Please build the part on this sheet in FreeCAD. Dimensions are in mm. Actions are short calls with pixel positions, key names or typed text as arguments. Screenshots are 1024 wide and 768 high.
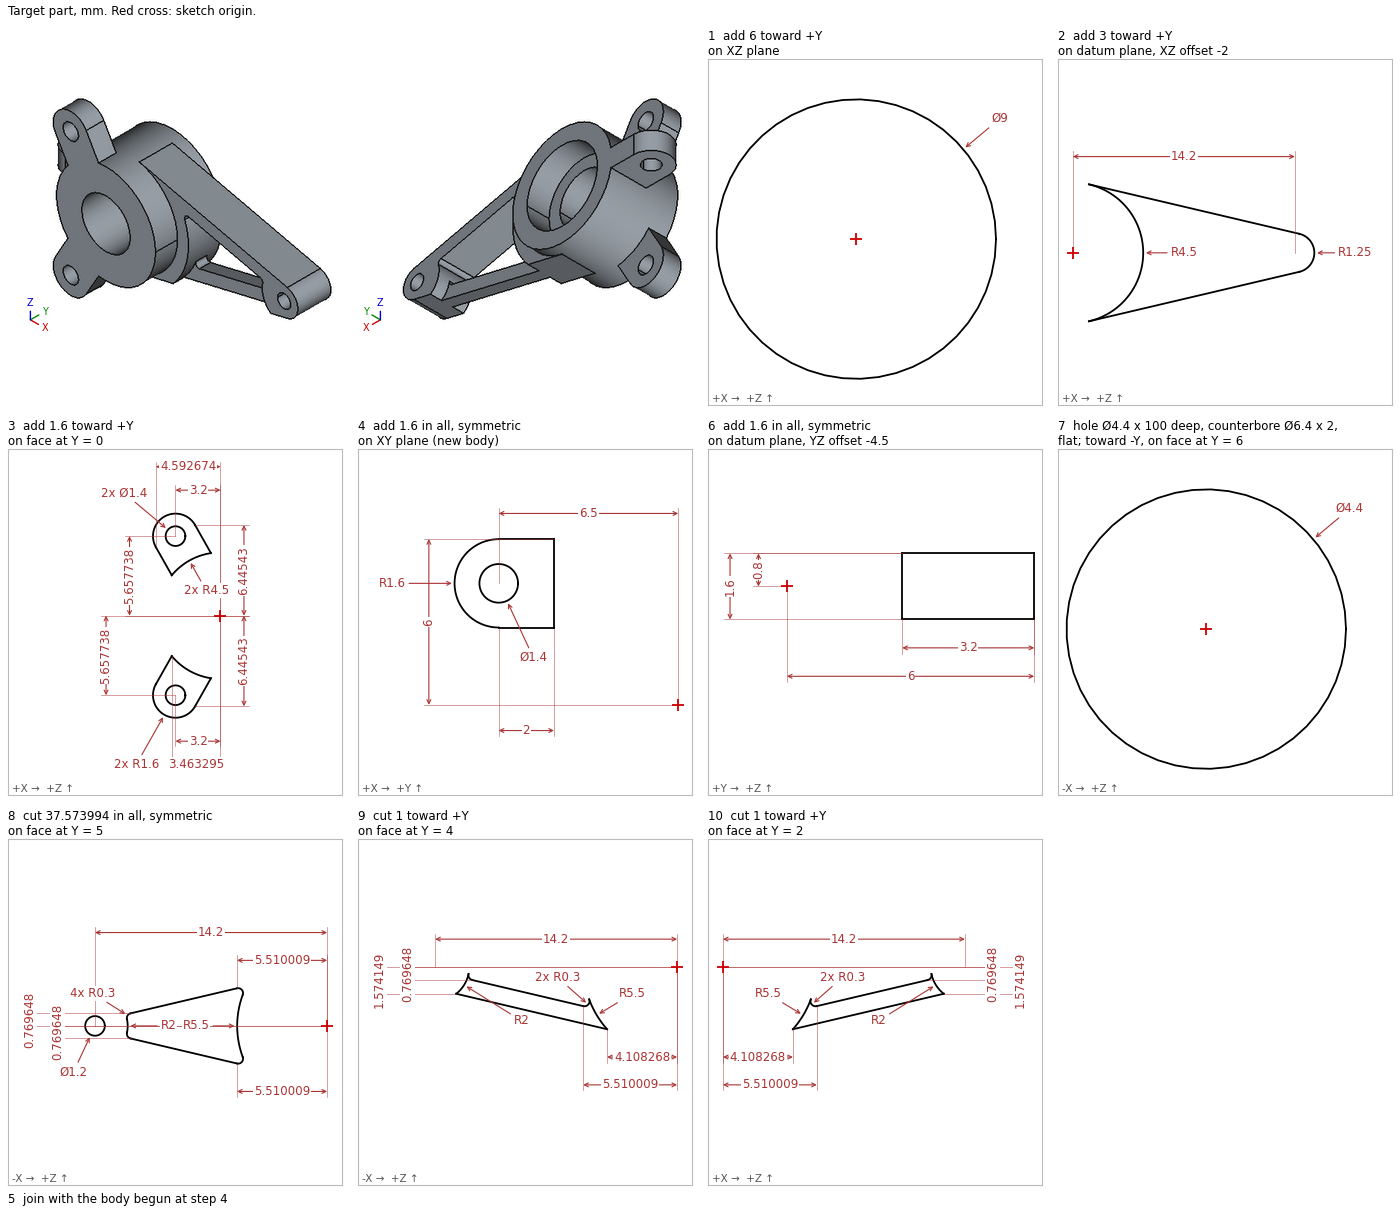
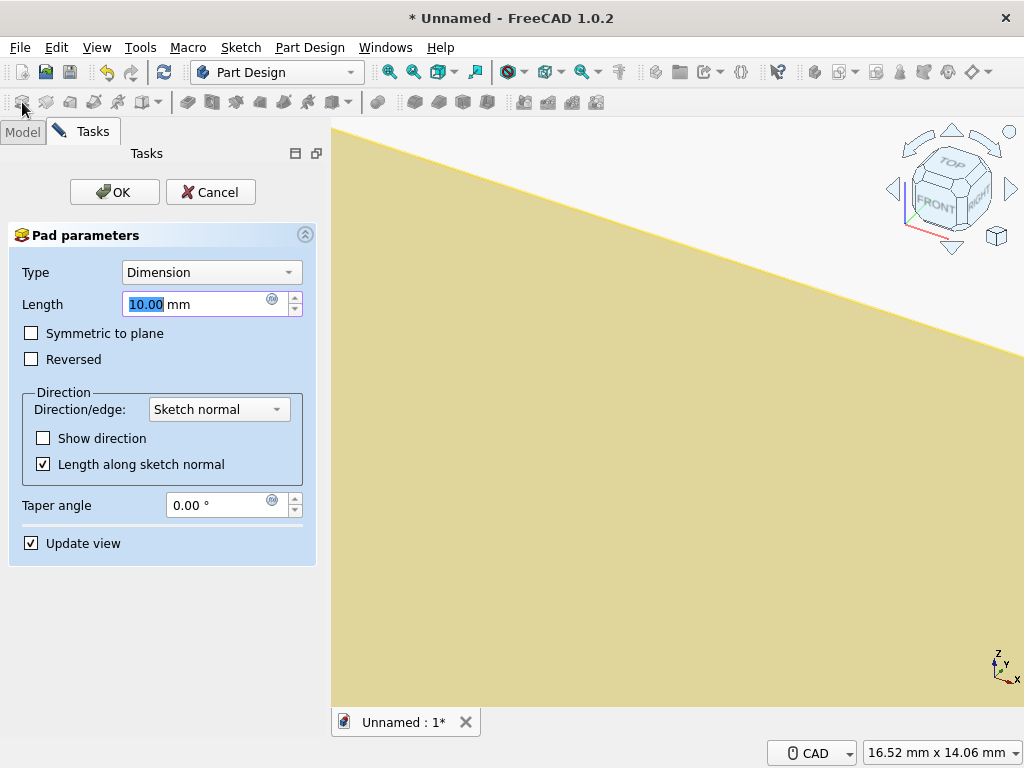
text(3)
key(Tab)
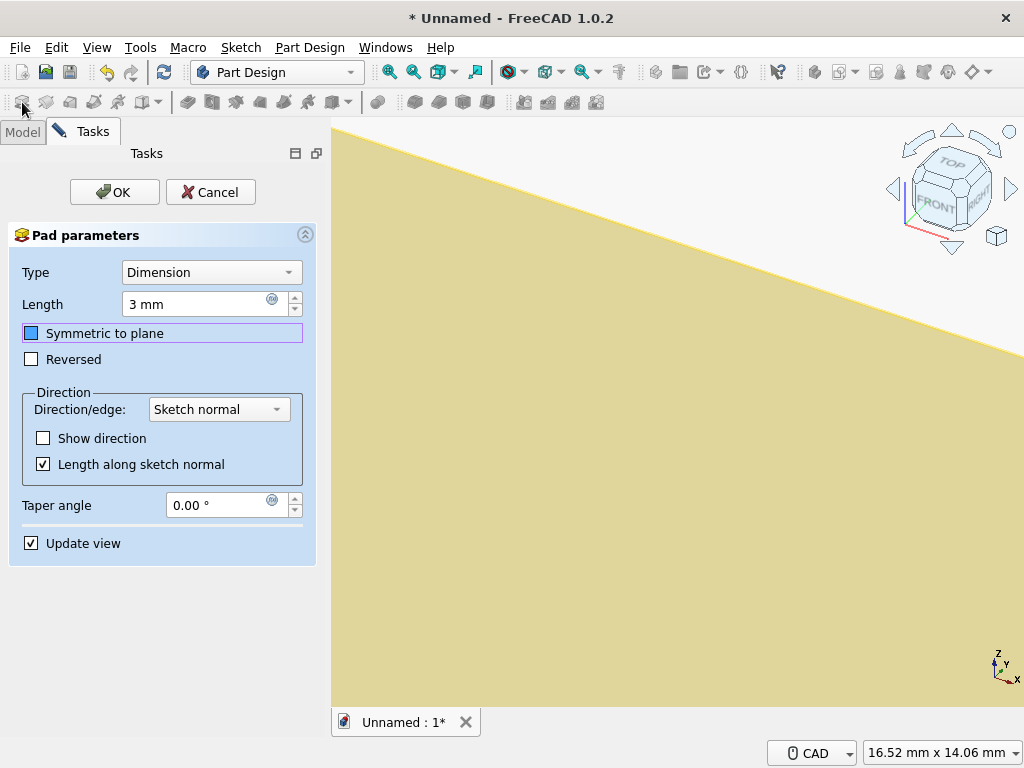
click(30, 359)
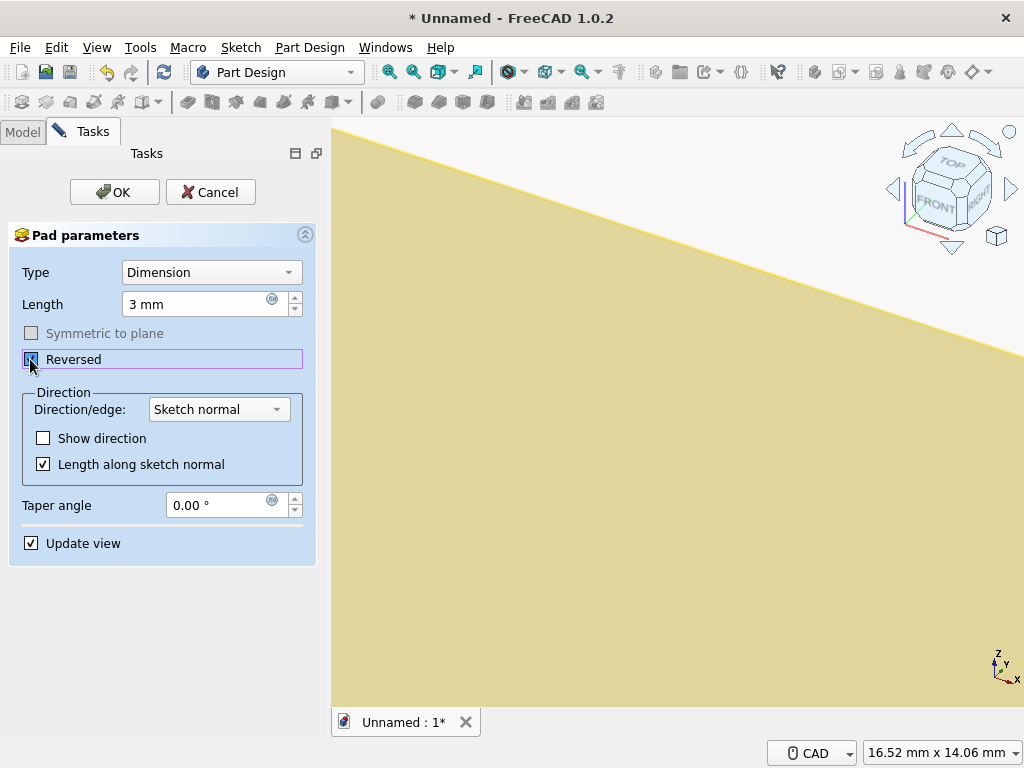
click(115, 192)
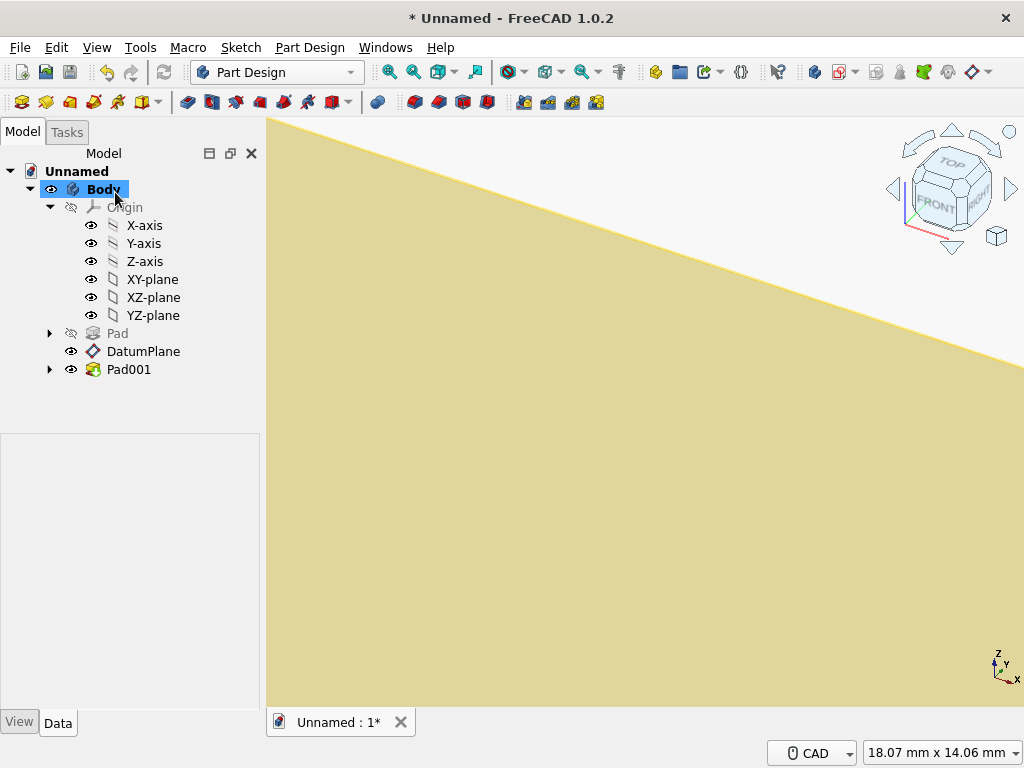
click(116, 351)
key(space)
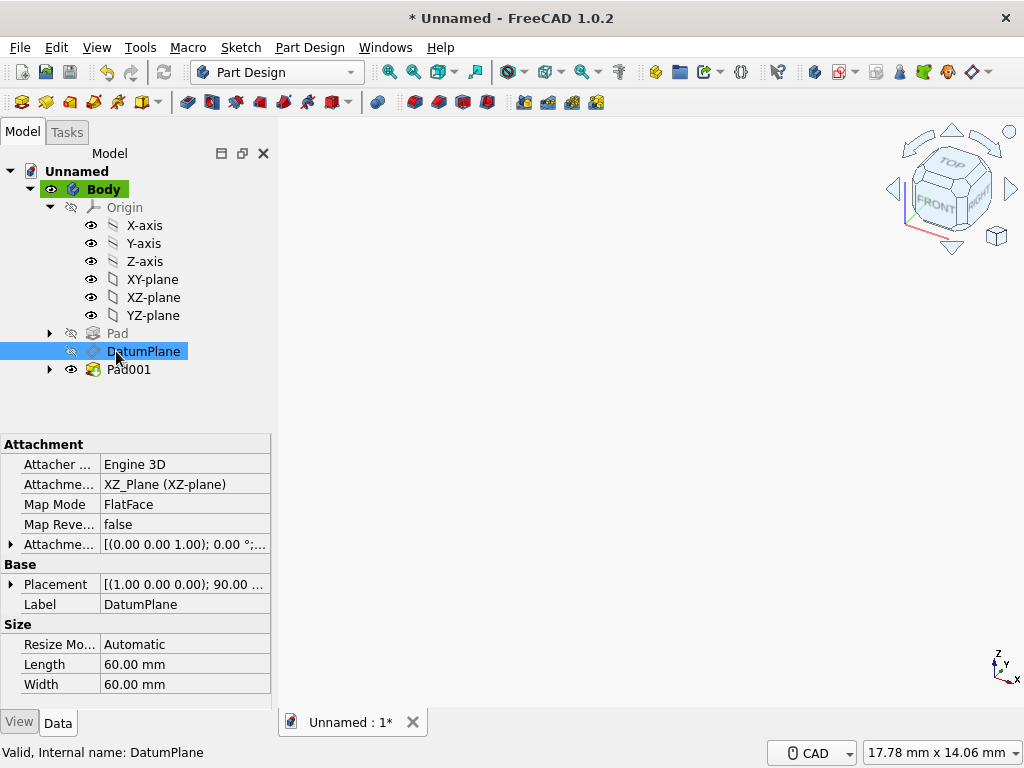
key(v)
key(f)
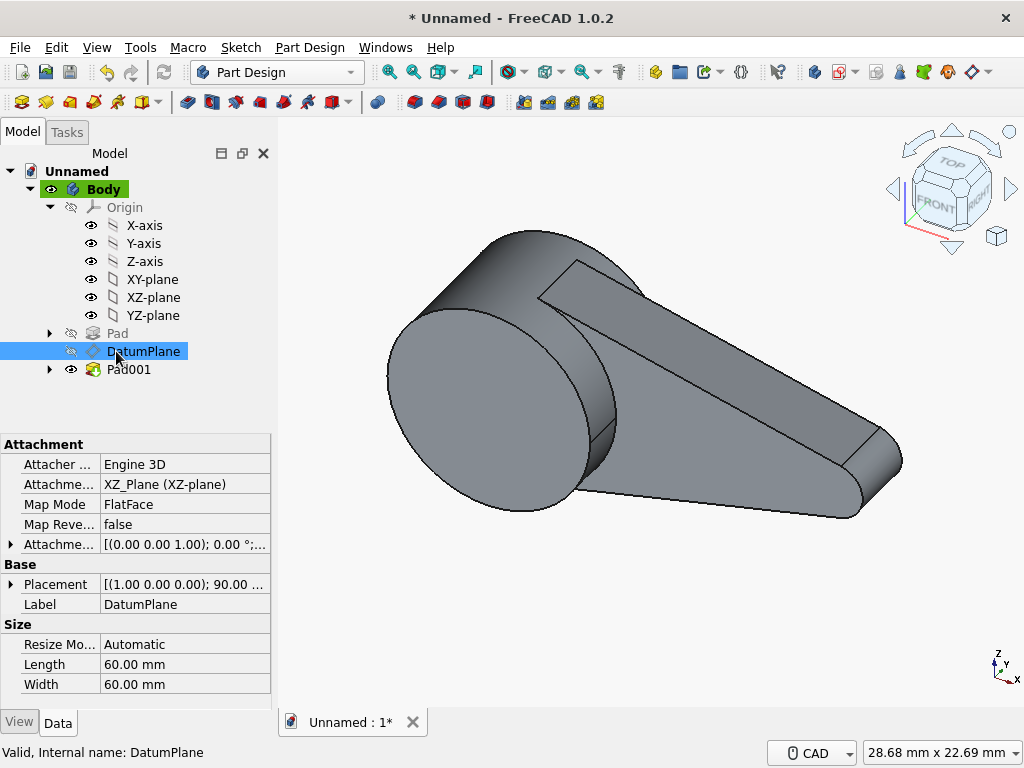
click(489, 409)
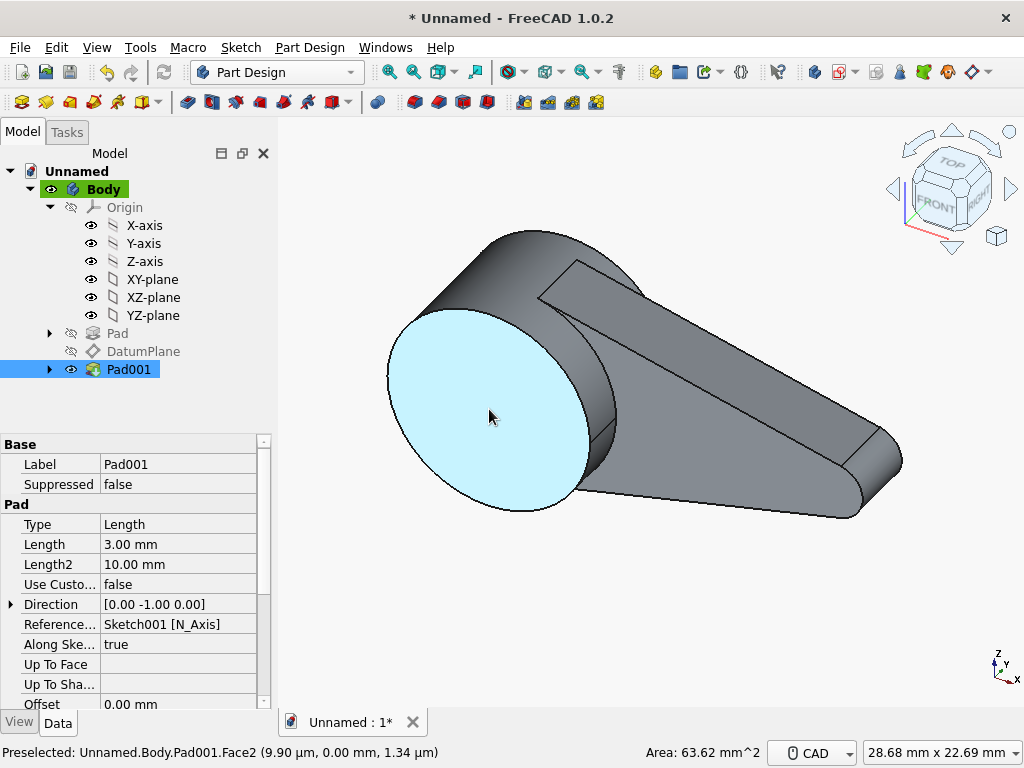
click(840, 72)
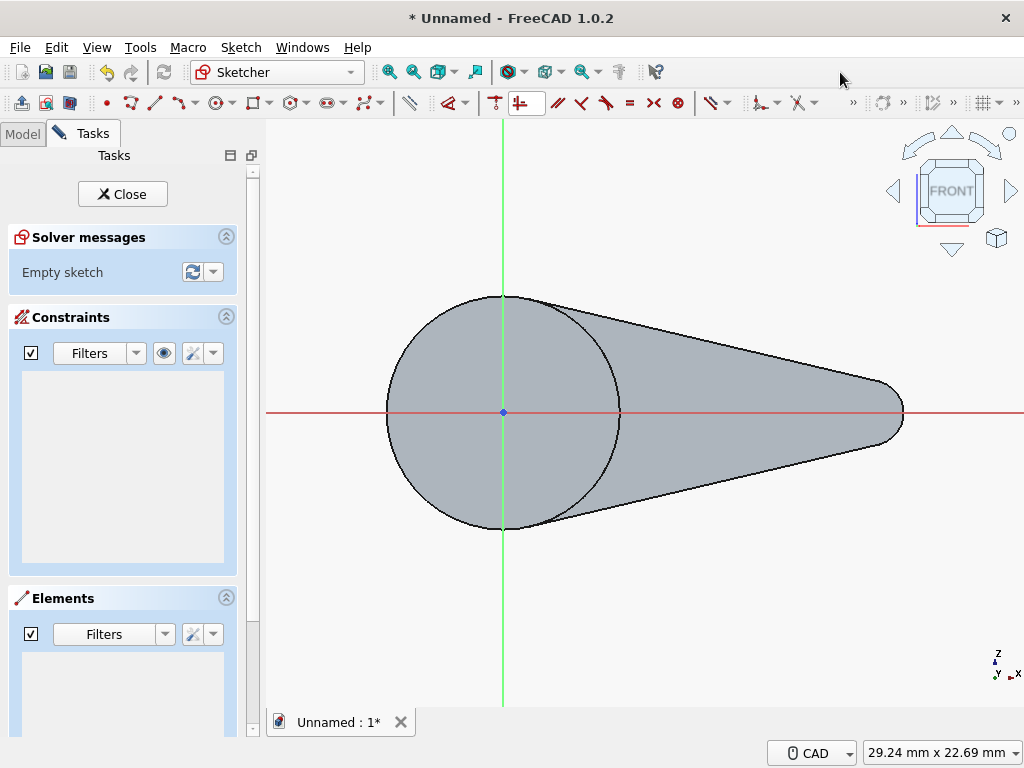
key(g)
key(l)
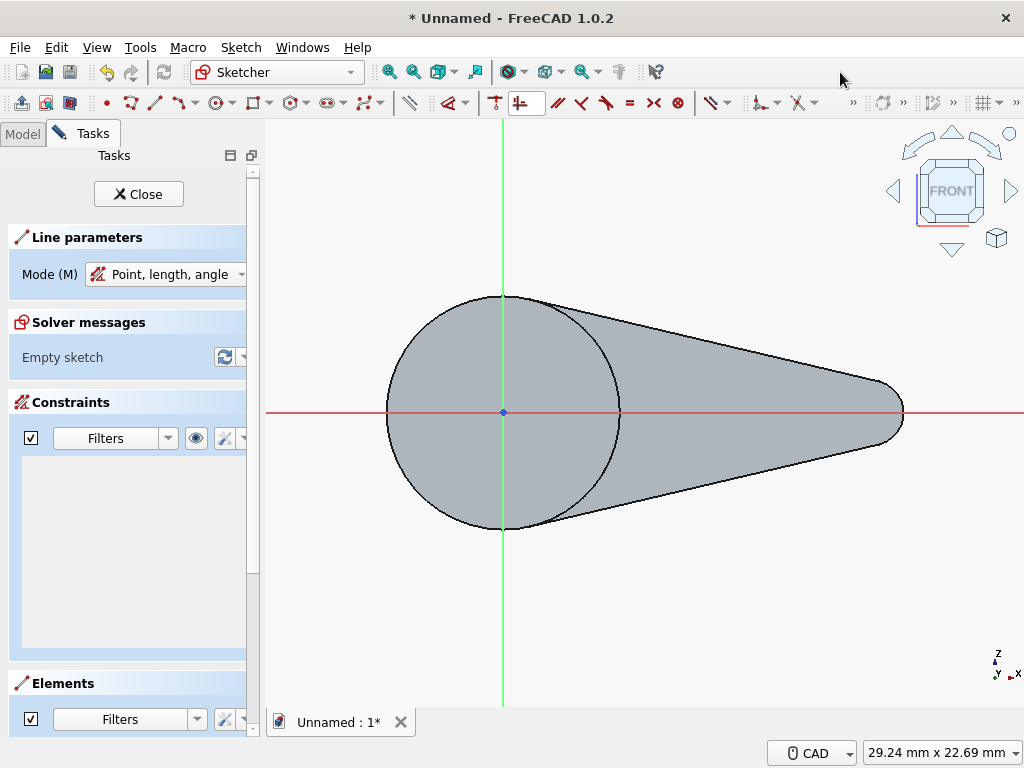
click(486, 298)
click(456, 246)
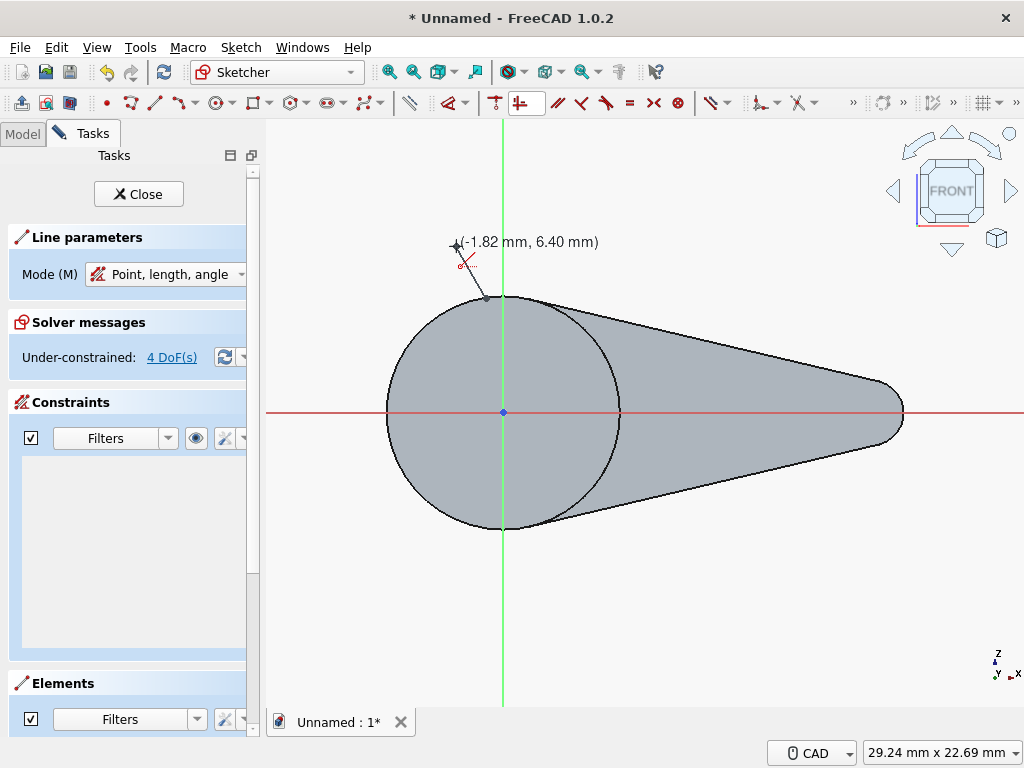
click(384, 287)
click(413, 339)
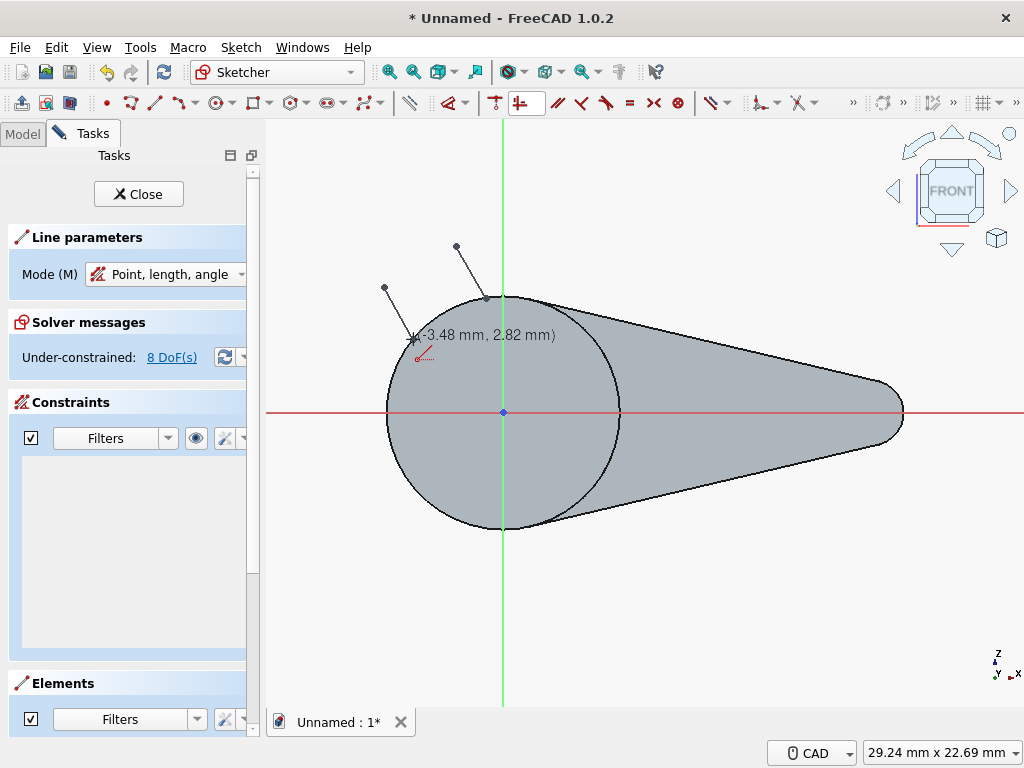
key(g)
key(3)
key(a)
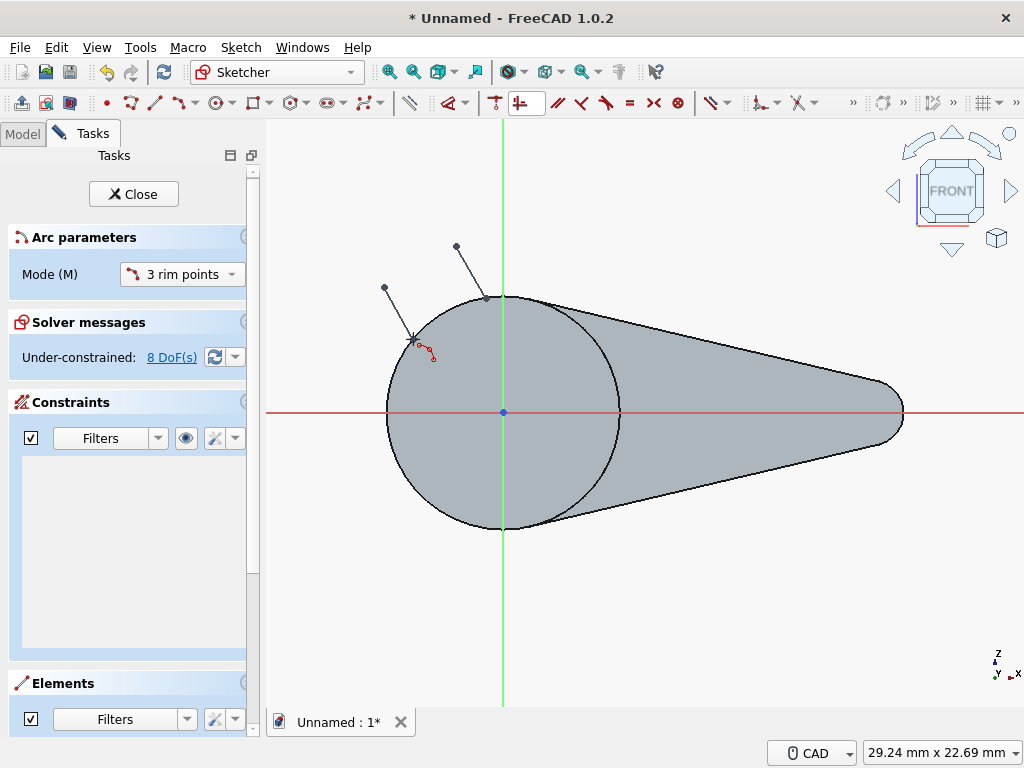
click(456, 247)
click(384, 288)
click(400, 230)